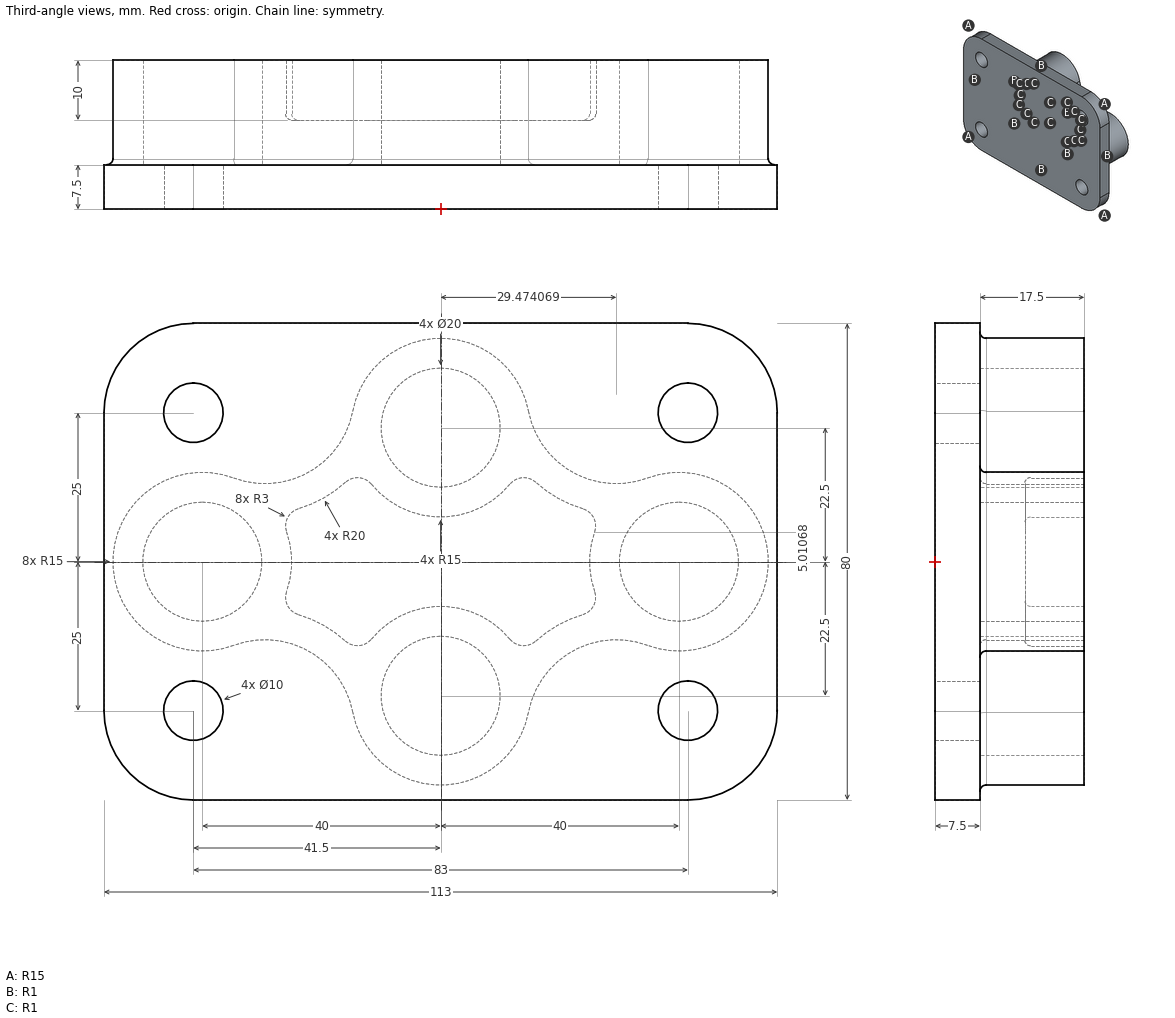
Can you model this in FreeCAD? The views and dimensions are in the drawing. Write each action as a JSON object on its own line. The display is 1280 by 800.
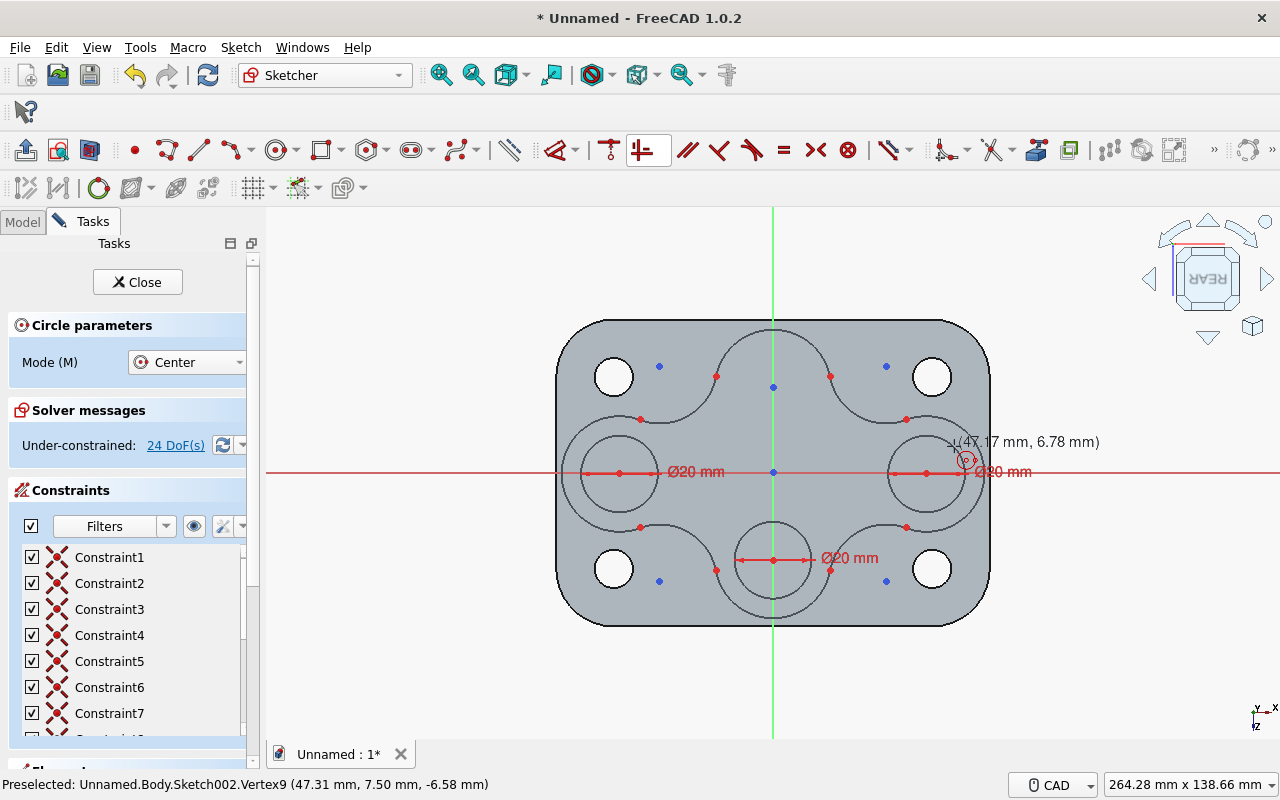
{"action": "left_click", "coordinate": [773, 387]}
{"action": "mouse_move", "coordinate": [800, 360]}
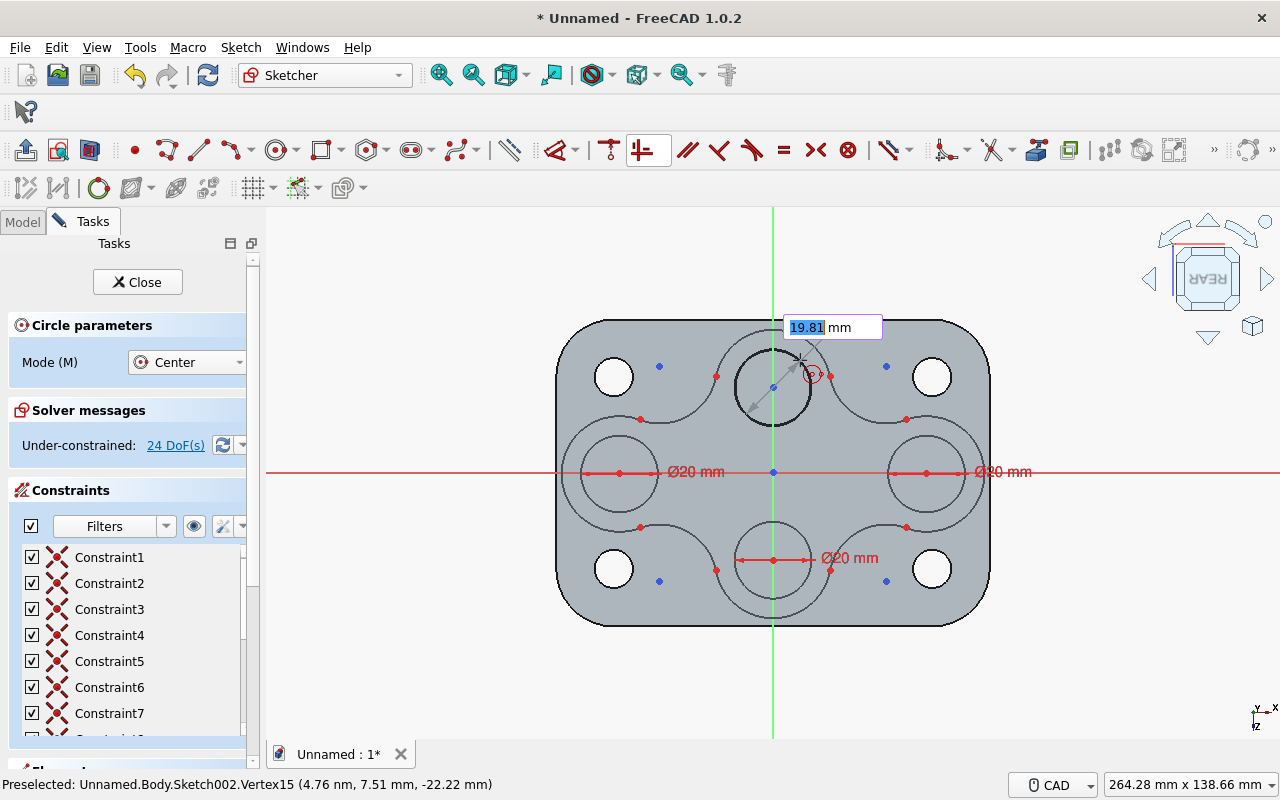
{"action": "type", "text": "20"}
{"action": "key", "text": "Return"}
{"action": "key", "text": "Escape"}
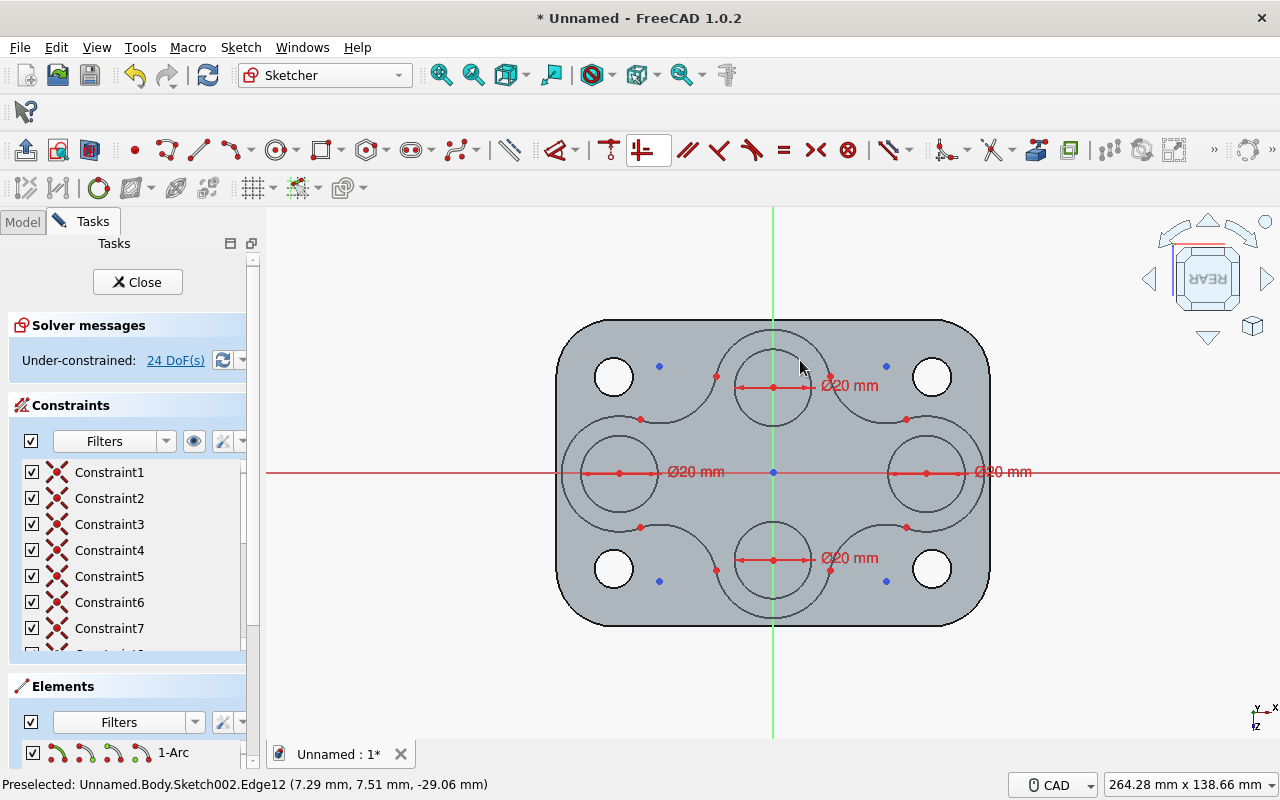
{"action": "left_click", "coordinate": [742, 610]}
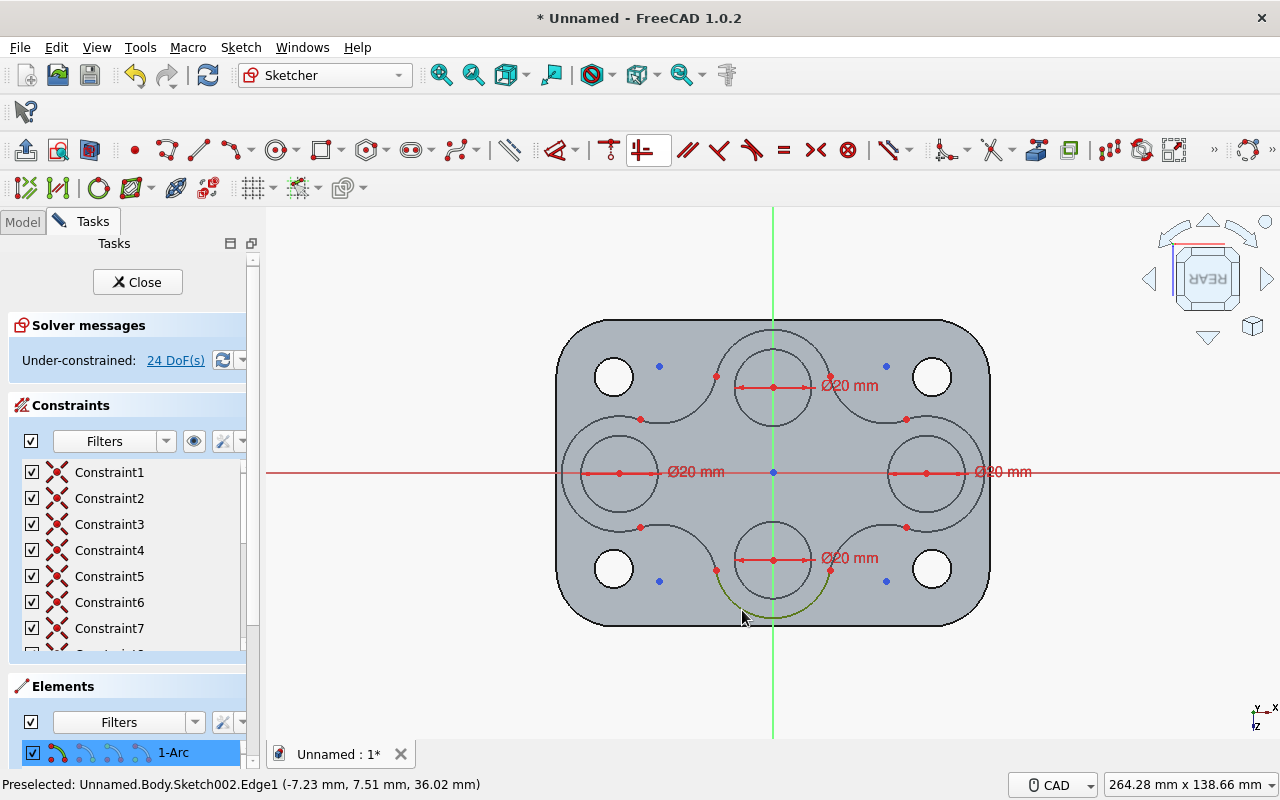
{"action": "left_click", "coordinate": [877, 525]}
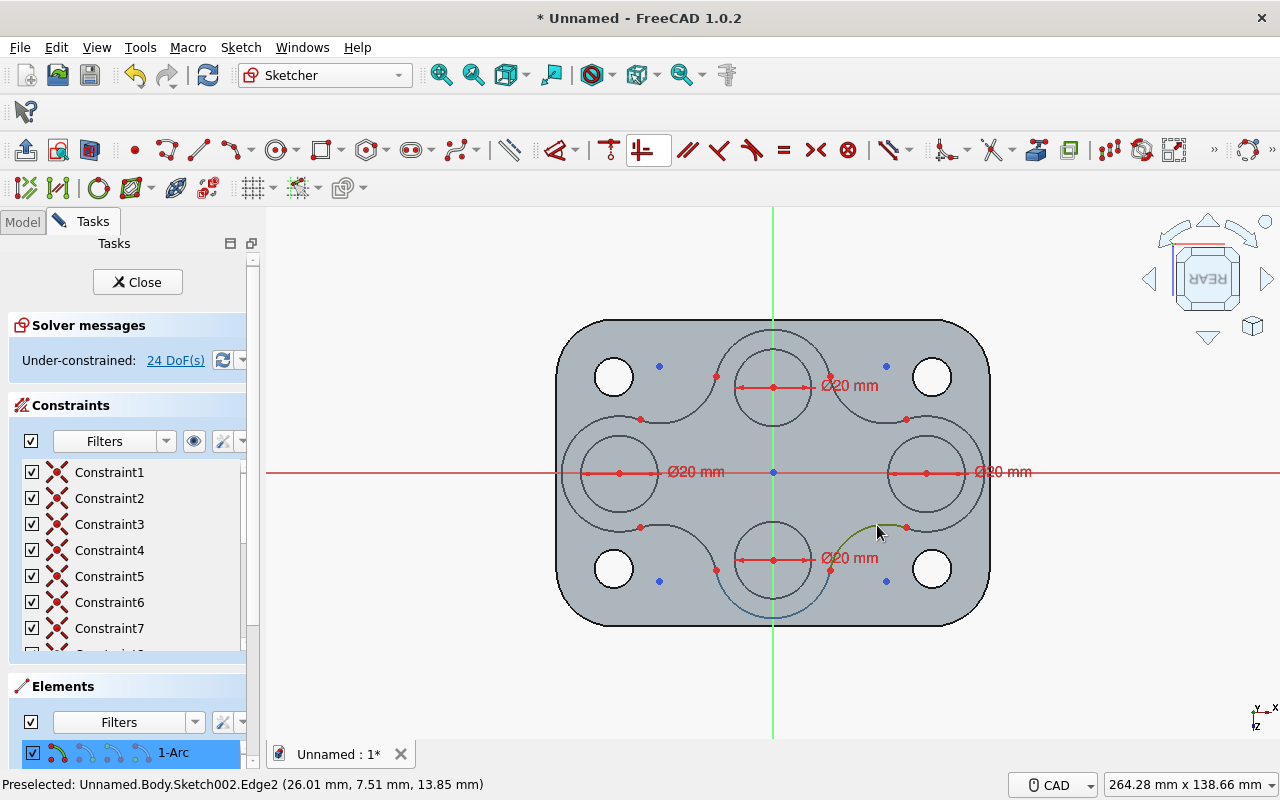
{"action": "key", "text": "t"}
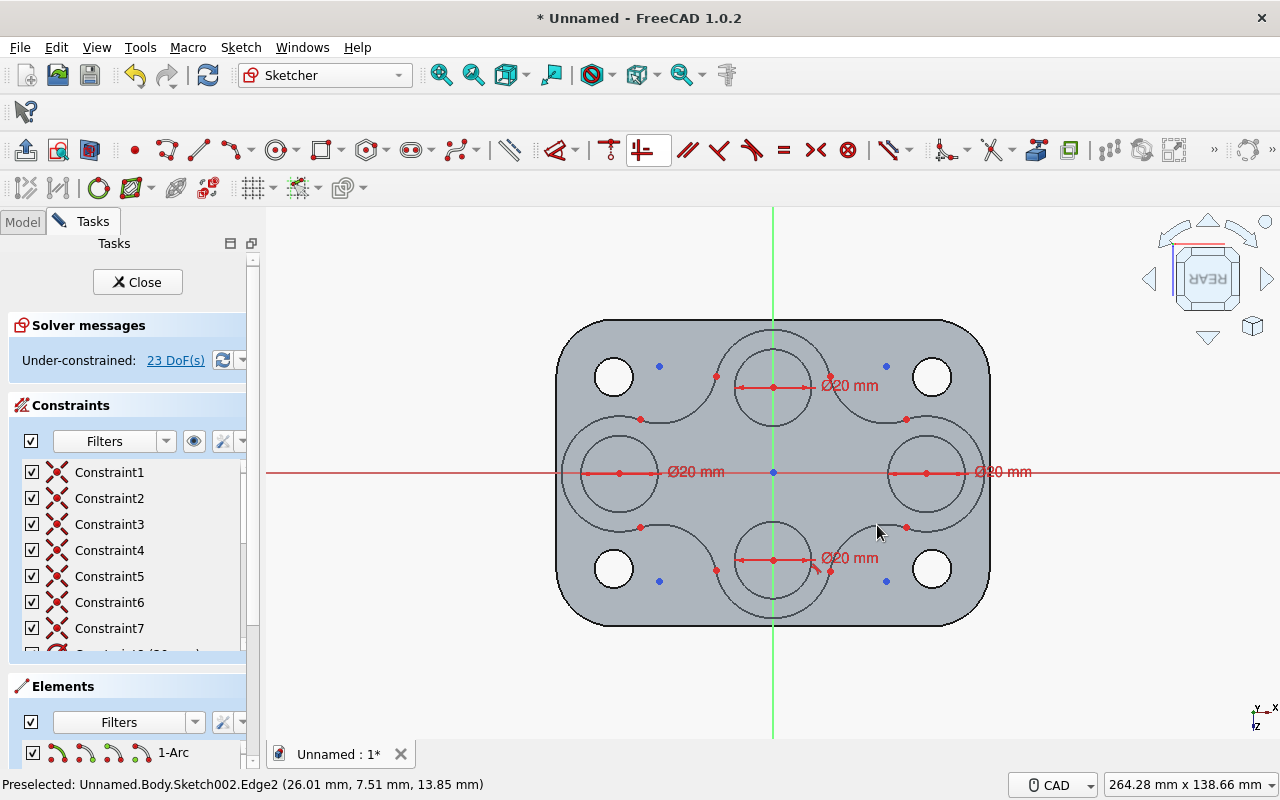
{"action": "left_click", "coordinate": [742, 610]}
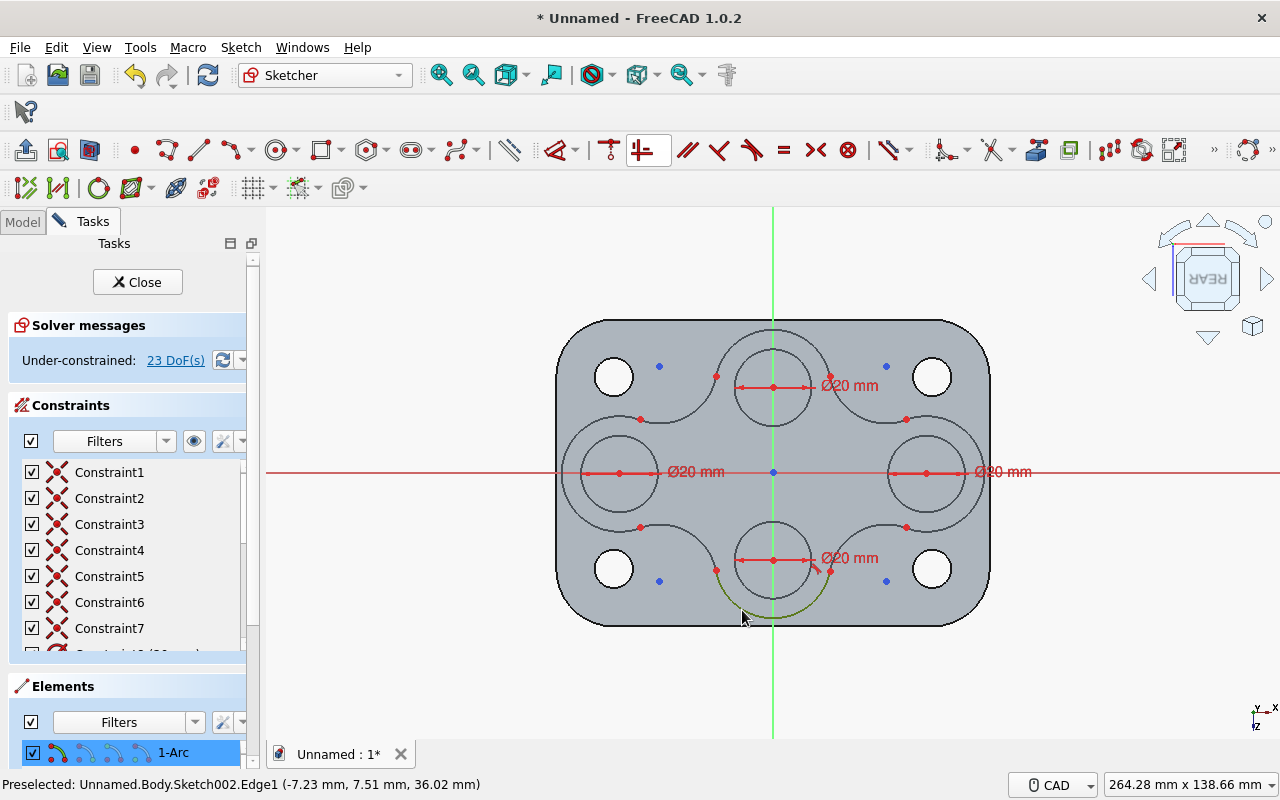
{"action": "left_click", "coordinate": [703, 544]}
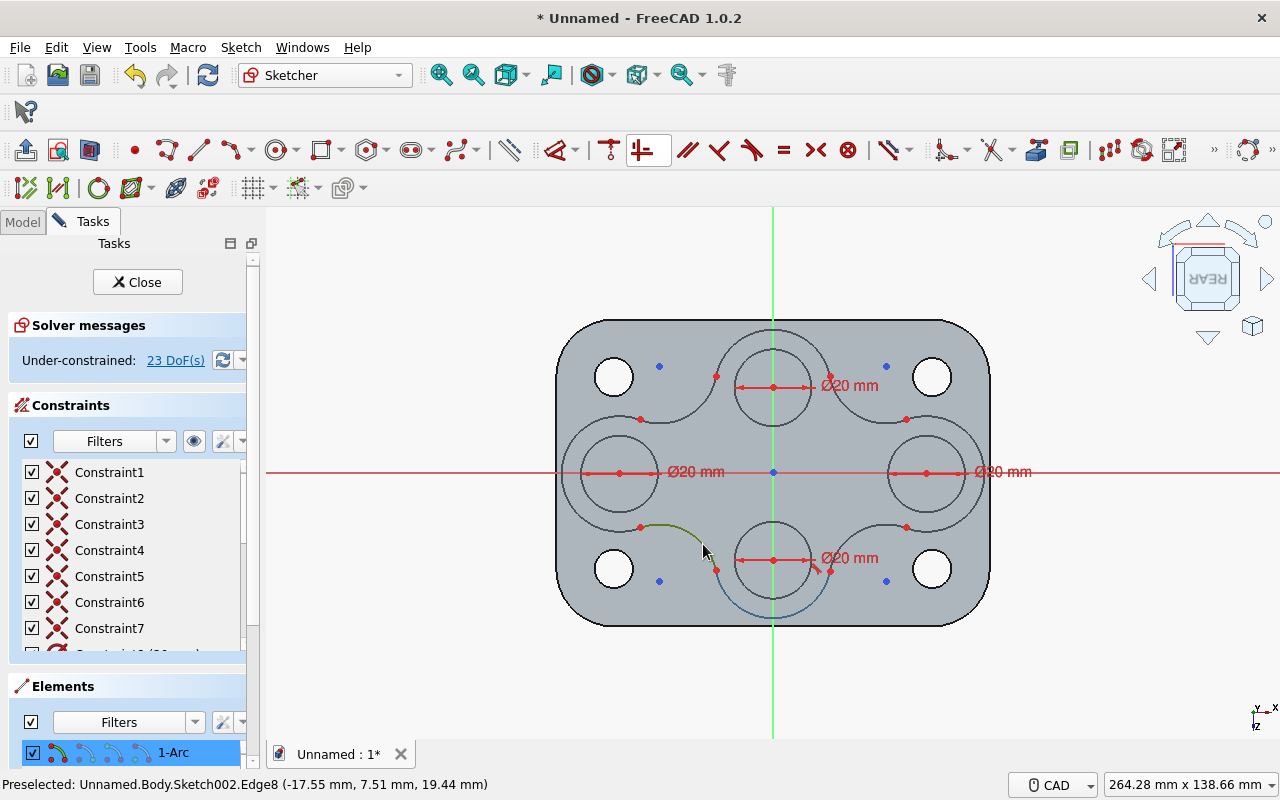
{"action": "key", "text": "t"}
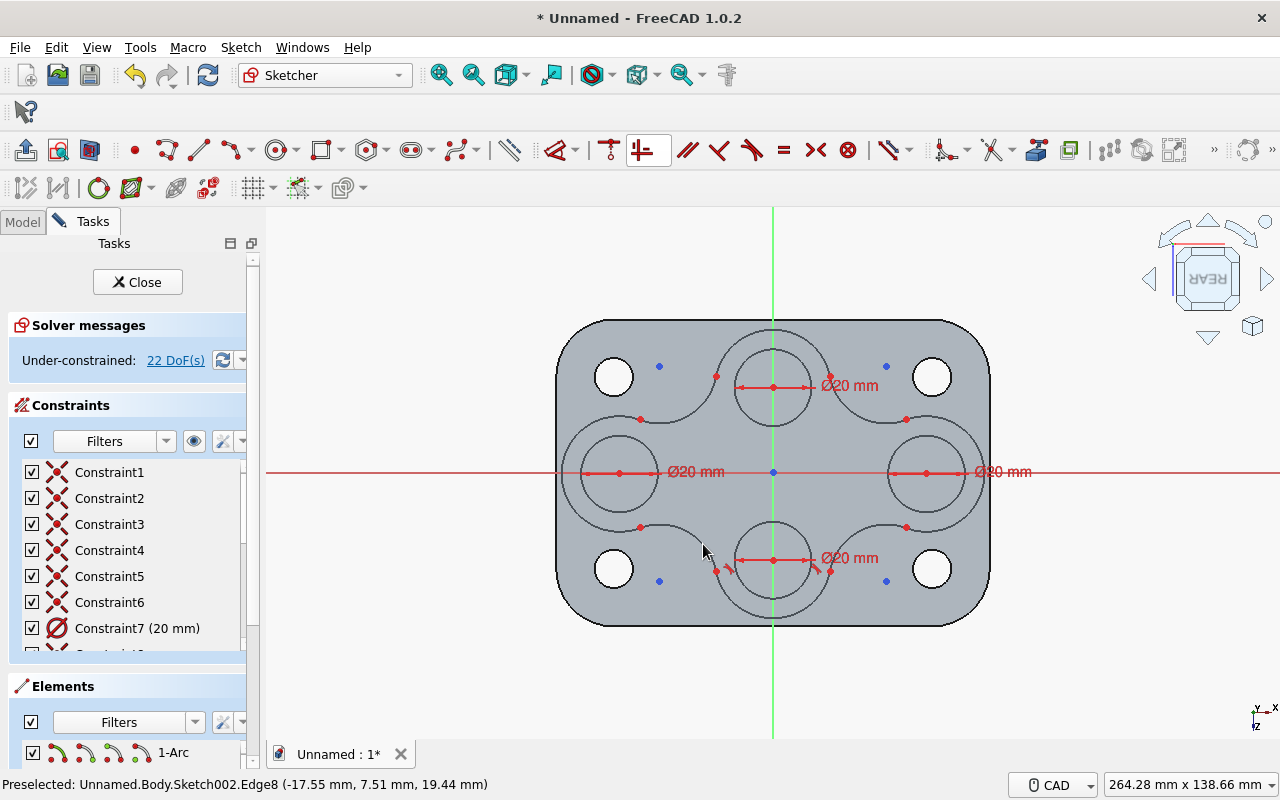
{"action": "left_click", "coordinate": [877, 525]}